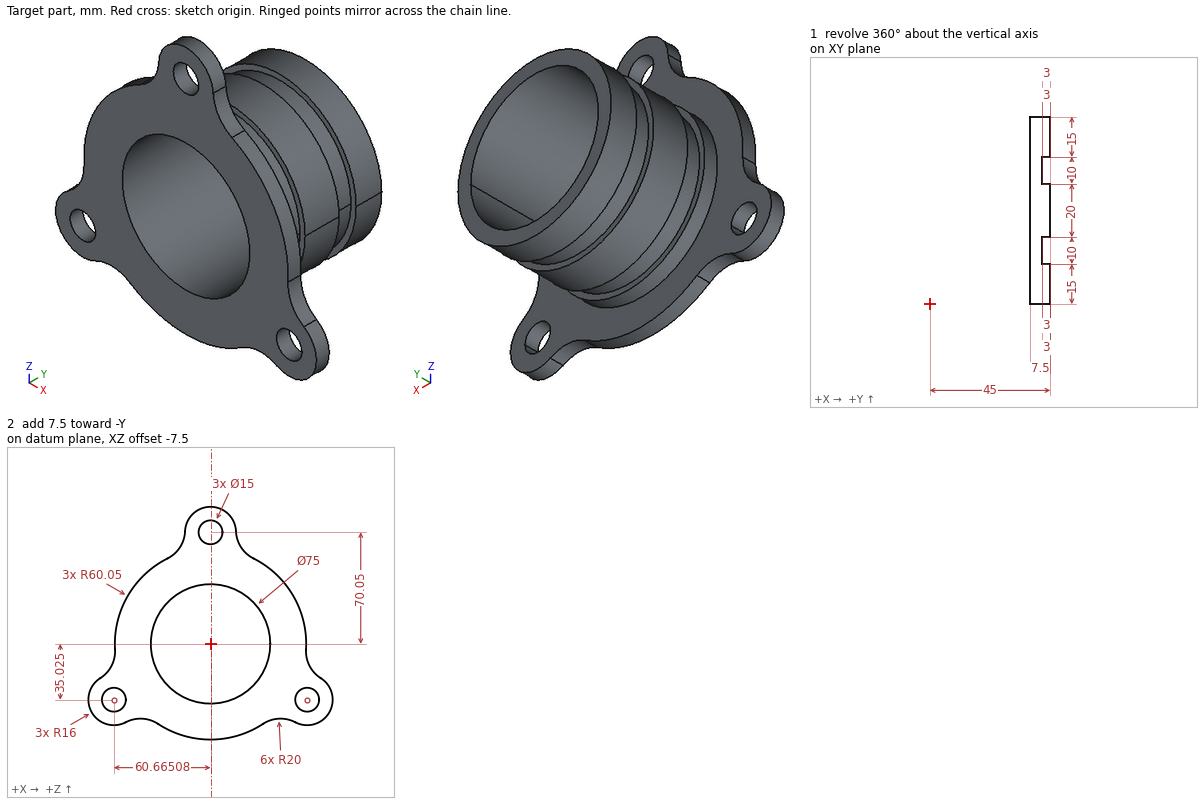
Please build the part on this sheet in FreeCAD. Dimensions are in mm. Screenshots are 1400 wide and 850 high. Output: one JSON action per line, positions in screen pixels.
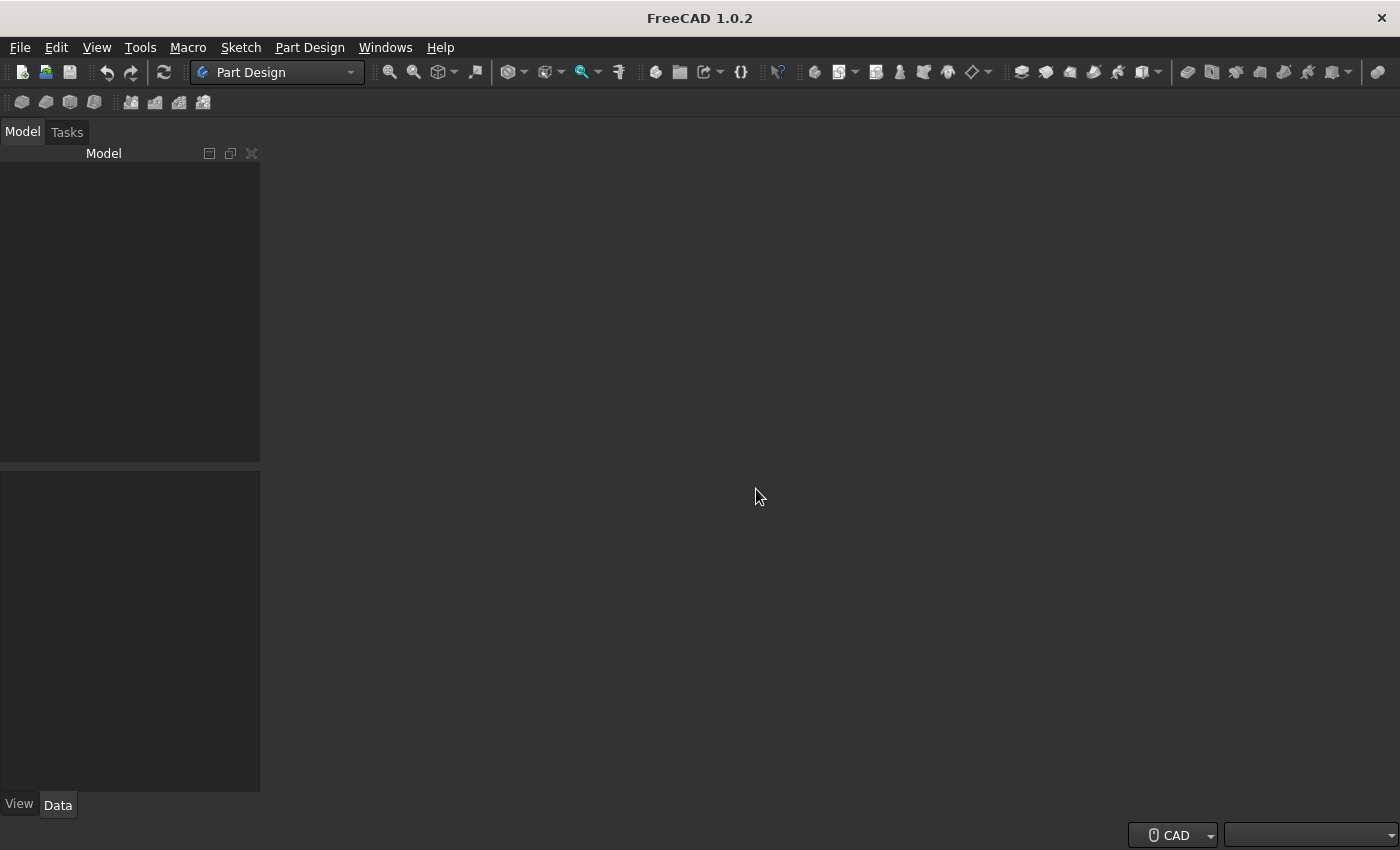
{"action": "left_click", "coordinate": [22, 72]}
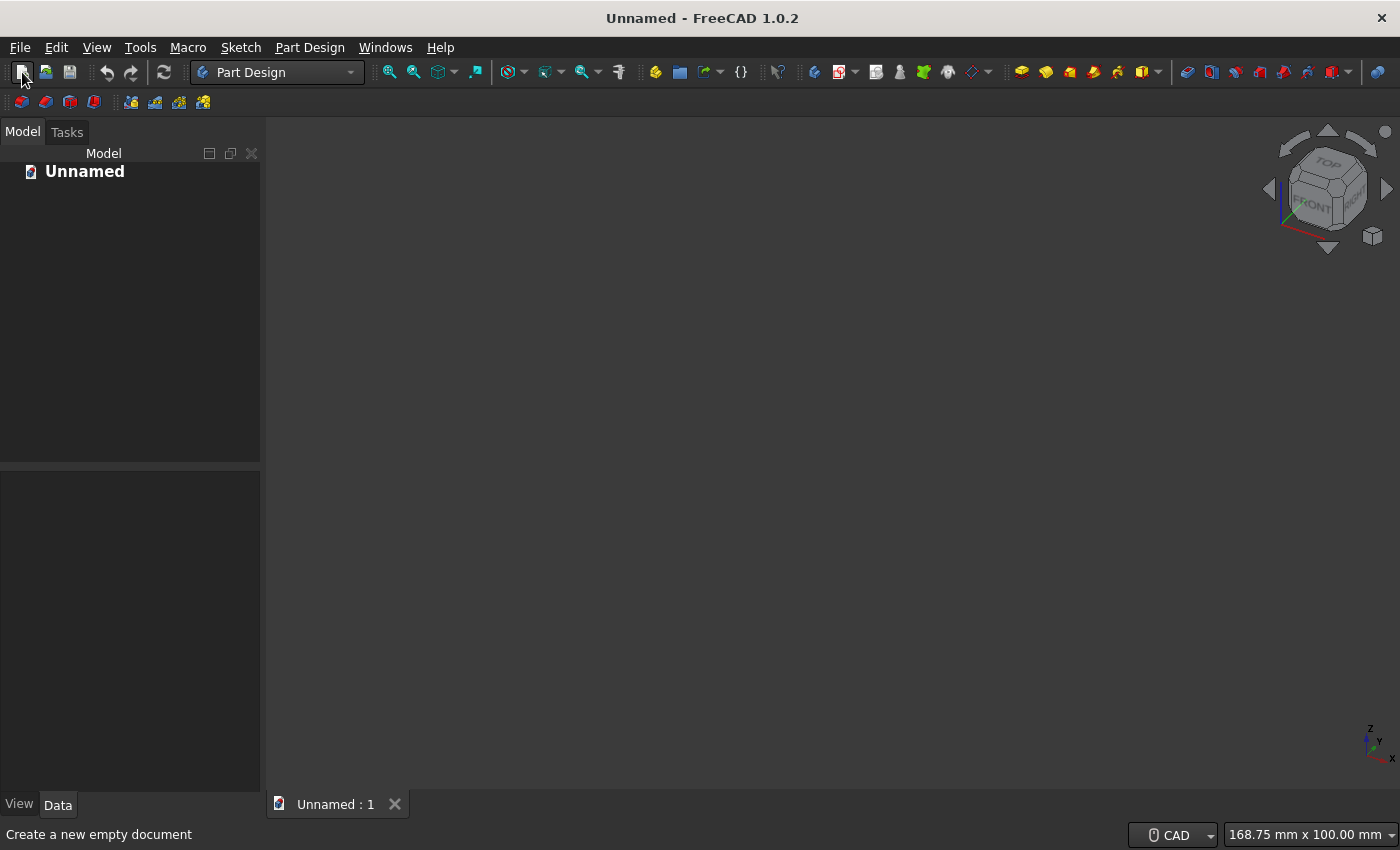
{"action": "left_click", "coordinate": [840, 72]}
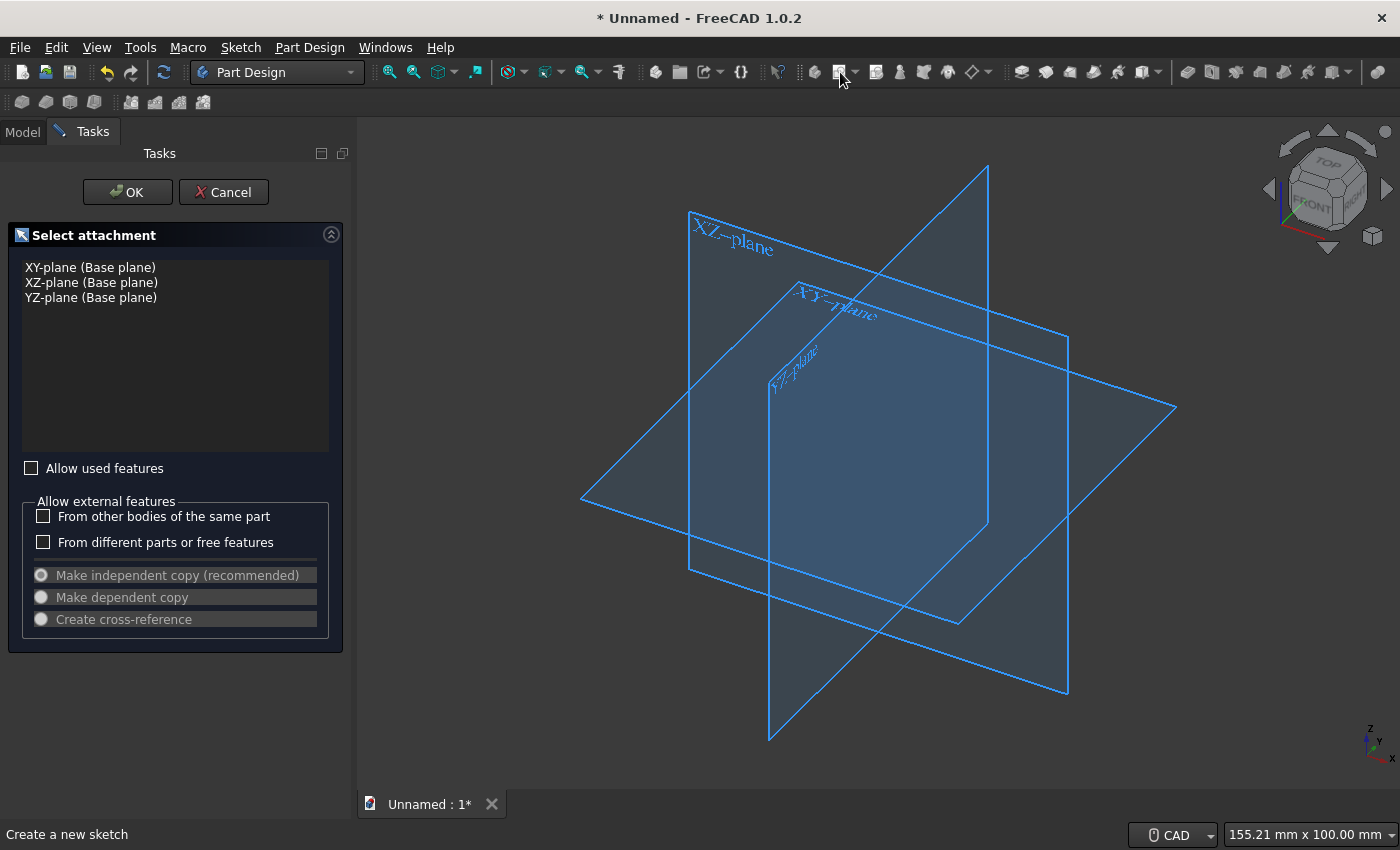
{"action": "left_click", "coordinate": [82, 268]}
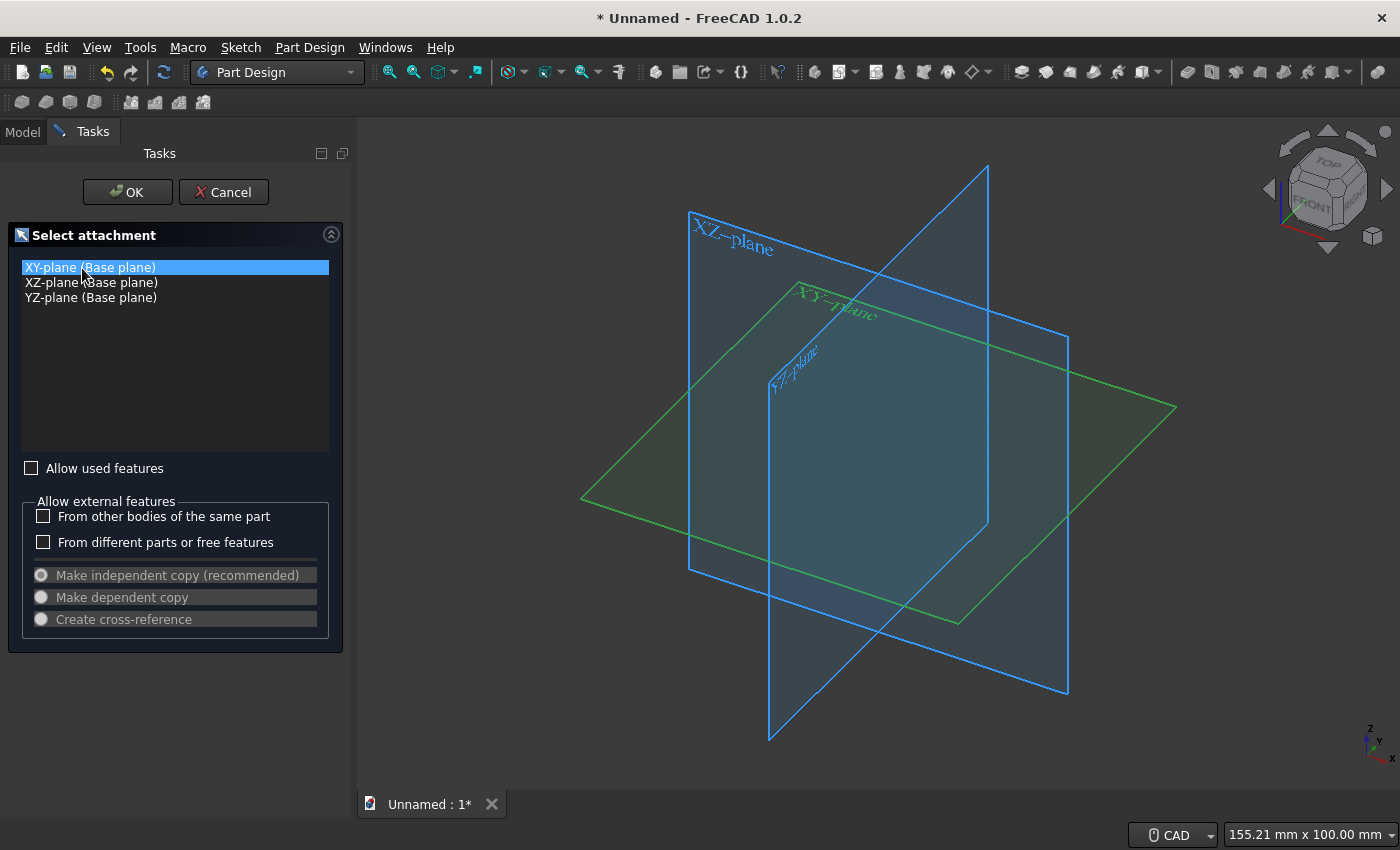
{"action": "left_click", "coordinate": [128, 192]}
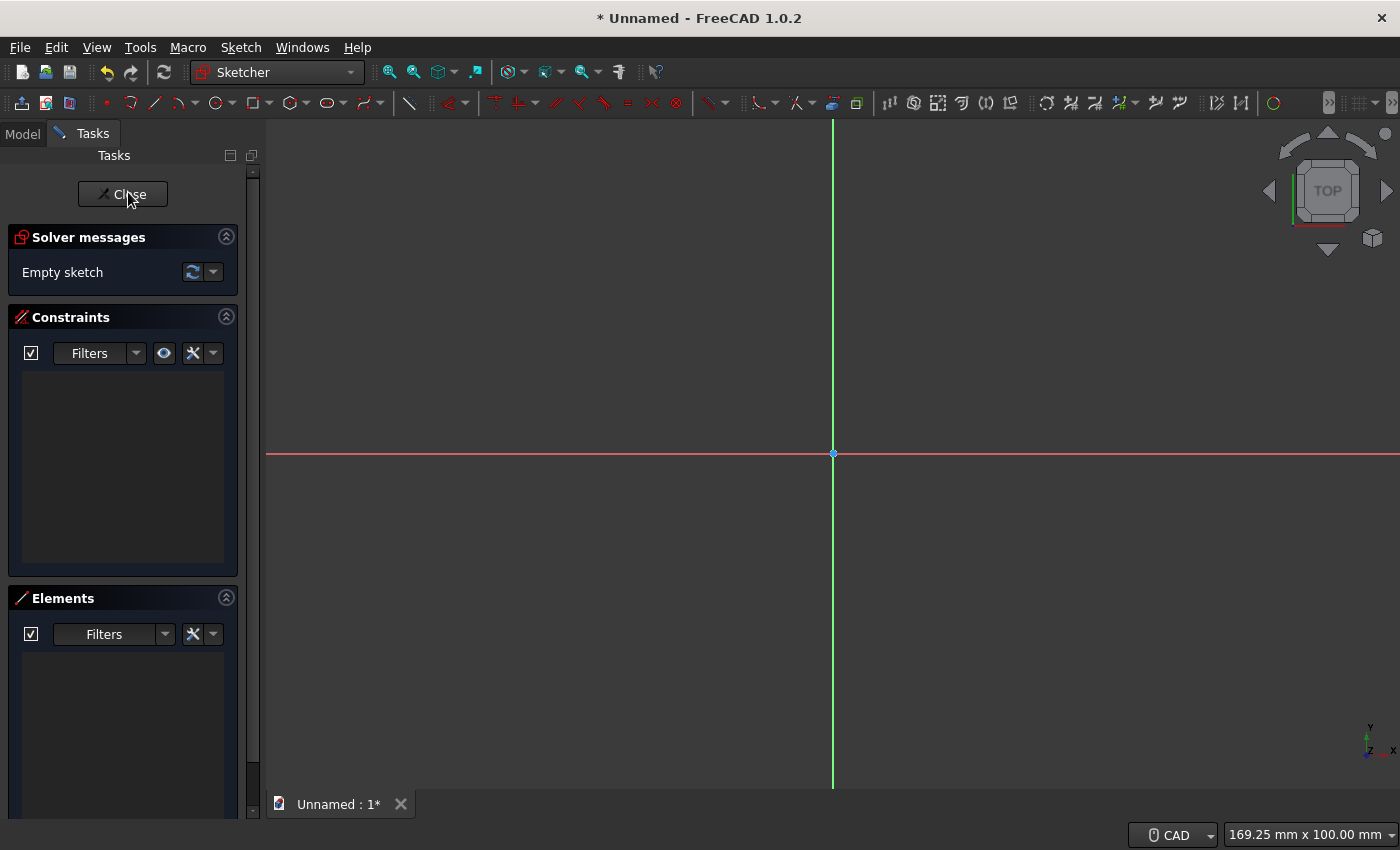
{"action": "scroll", "coordinate": [319, 761], "scroll_direction": "down", "scroll_amount": 2}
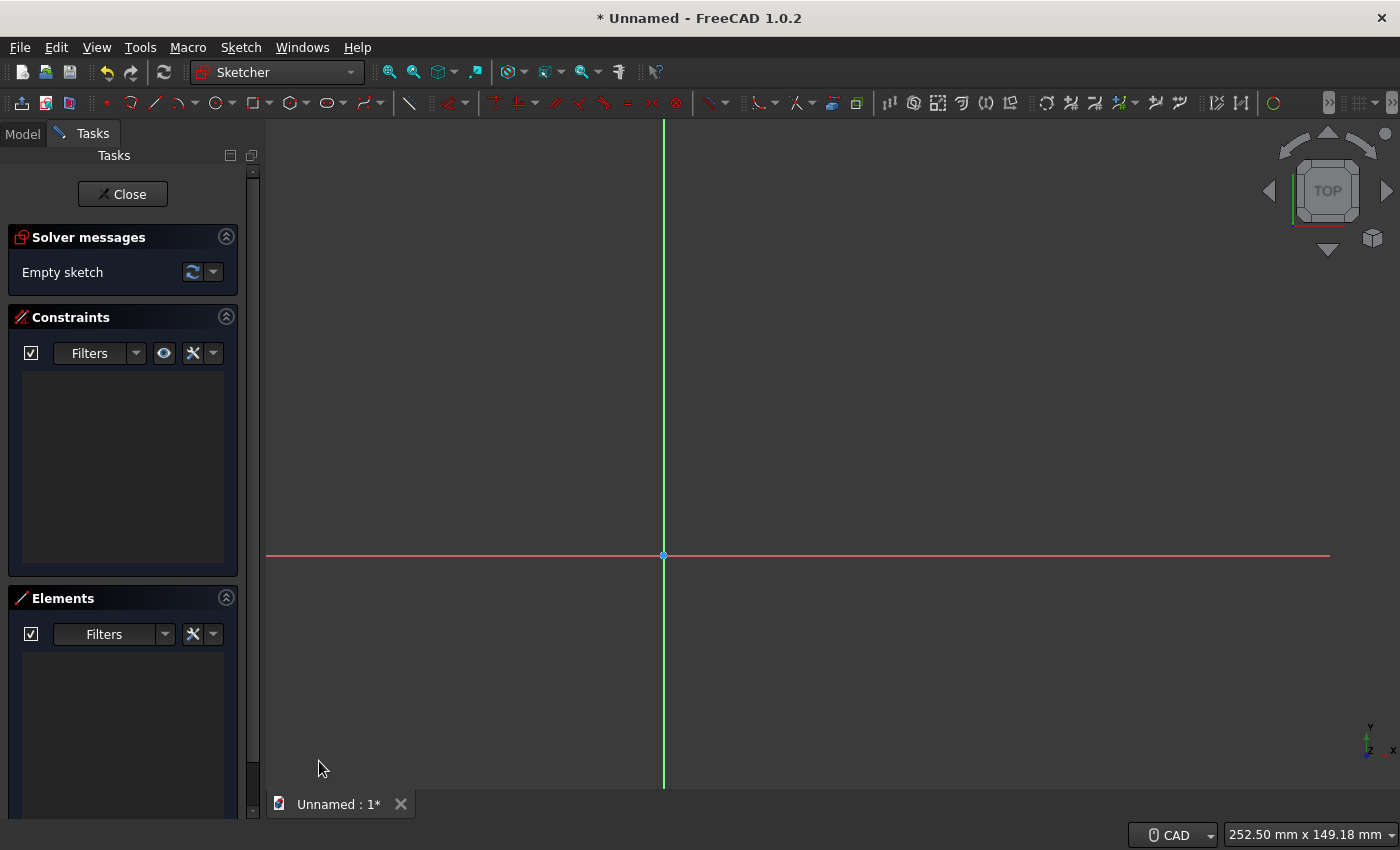
{"action": "scroll", "coordinate": [765, 285], "scroll_direction": "up", "scroll_amount": 2}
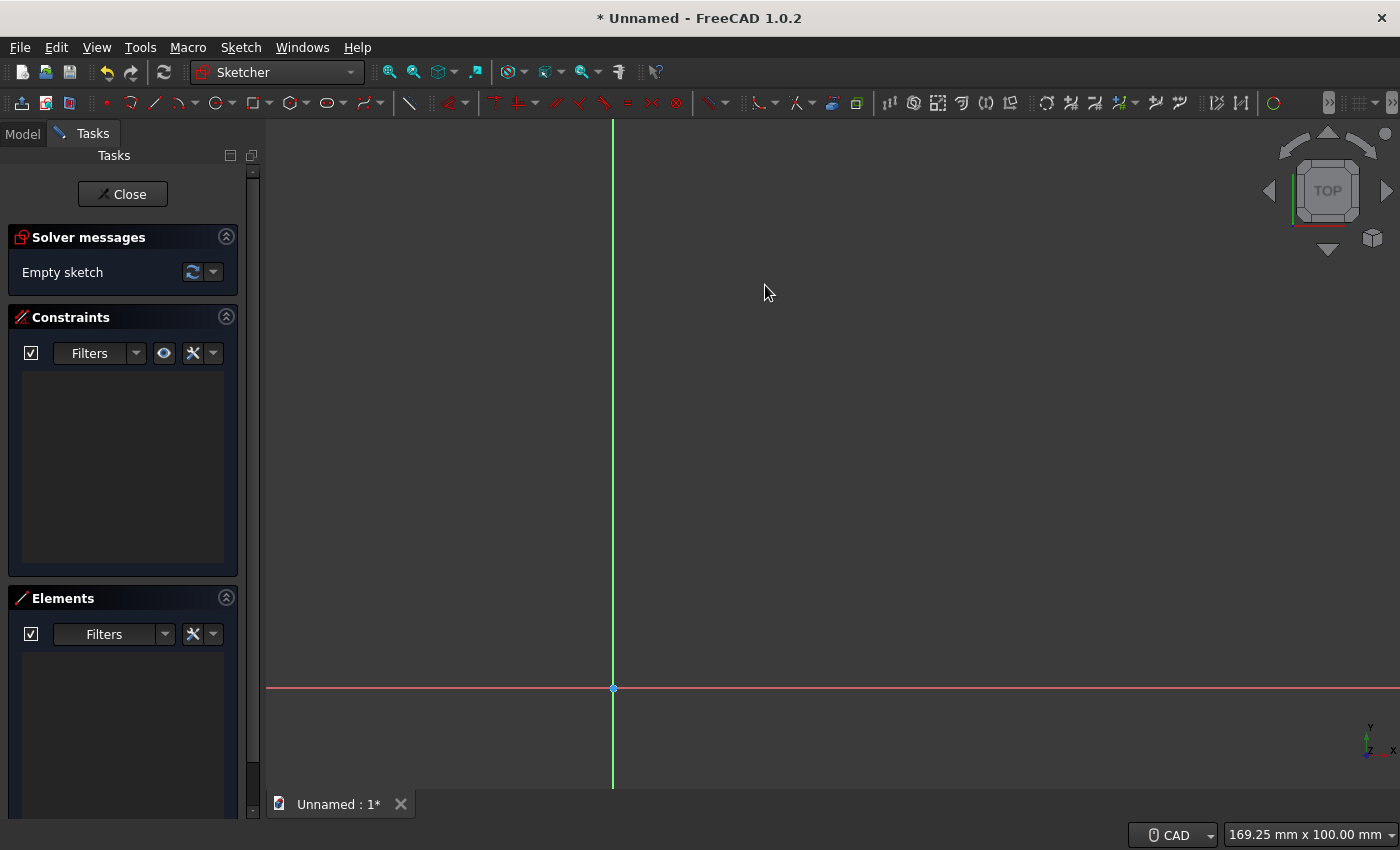
{"action": "key", "text": "g m"}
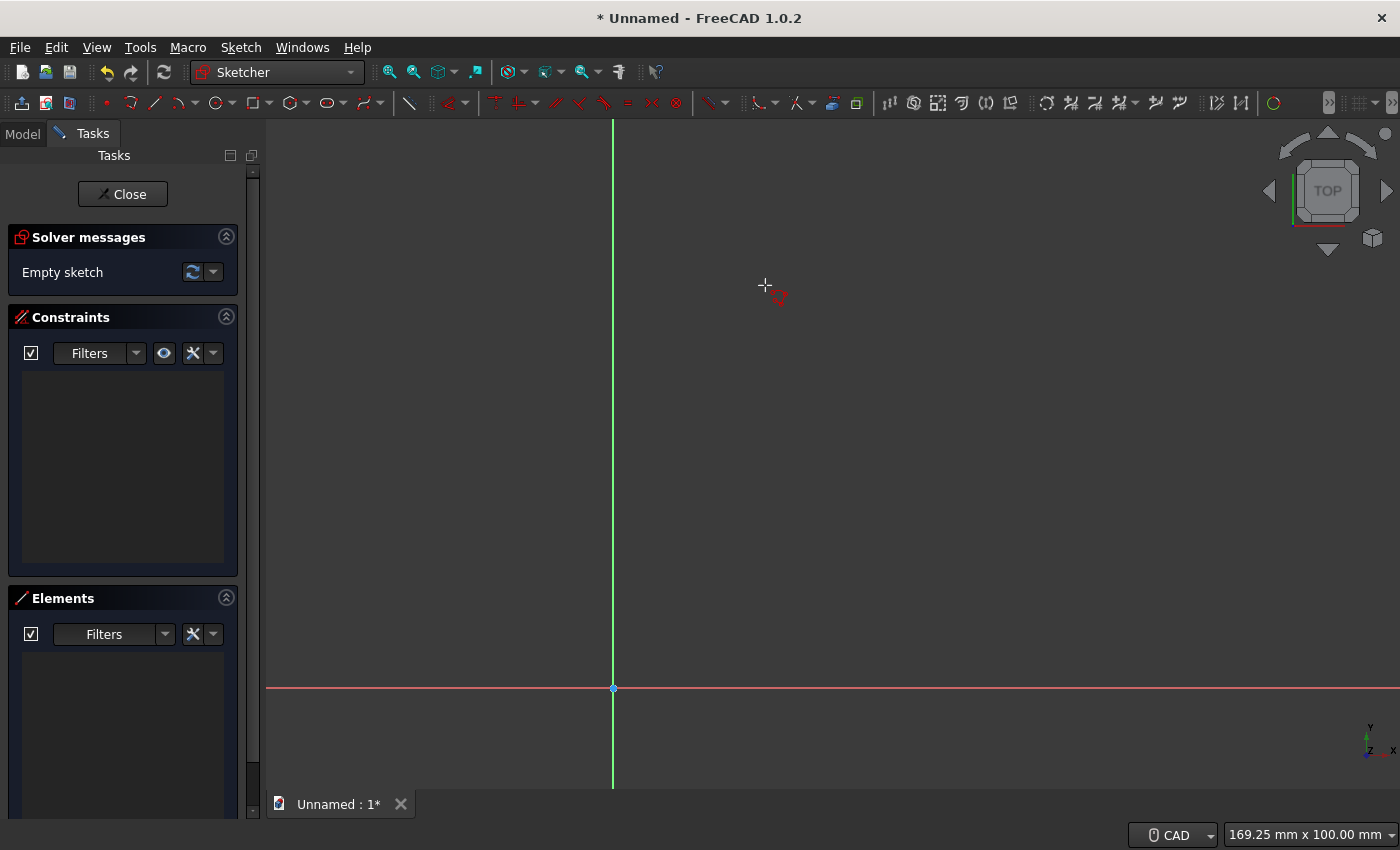
{"action": "left_click", "coordinate": [865, 688]}
{"action": "left_click", "coordinate": [915, 679]}
{"action": "left_click", "coordinate": [915, 588]}
{"action": "left_click", "coordinate": [895, 588]}
{"action": "left_click", "coordinate": [895, 521]}
{"action": "left_click", "coordinate": [915, 521]}
{"action": "left_click", "coordinate": [915, 387]}
{"action": "left_click", "coordinate": [895, 387]}
{"action": "left_click", "coordinate": [895, 320]}
{"action": "left_click", "coordinate": [915, 320]}
{"action": "left_click", "coordinate": [915, 219]}
{"action": "left_click", "coordinate": [865, 219]}
{"action": "left_click", "coordinate": [865, 688]}
{"action": "key", "text": "Escape"}
{"action": "key", "text": "Escape"}